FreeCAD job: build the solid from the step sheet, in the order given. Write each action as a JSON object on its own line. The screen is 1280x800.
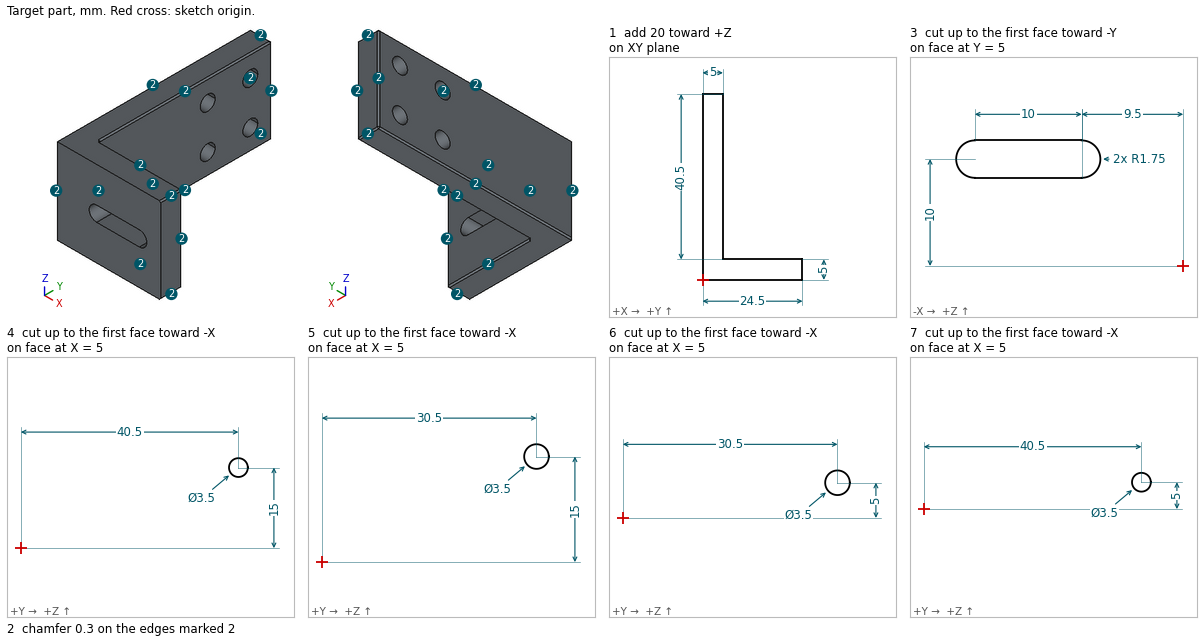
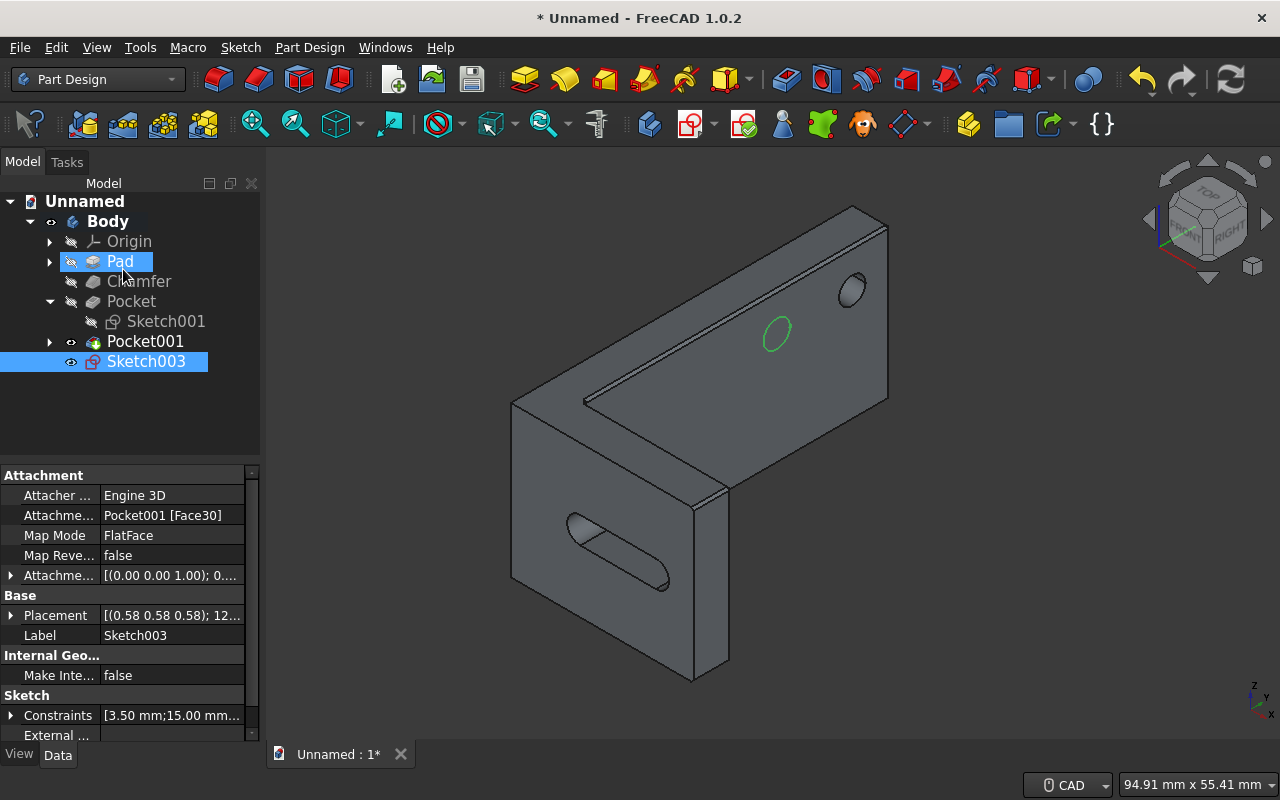
{"action": "left_click", "coordinate": [788, 80]}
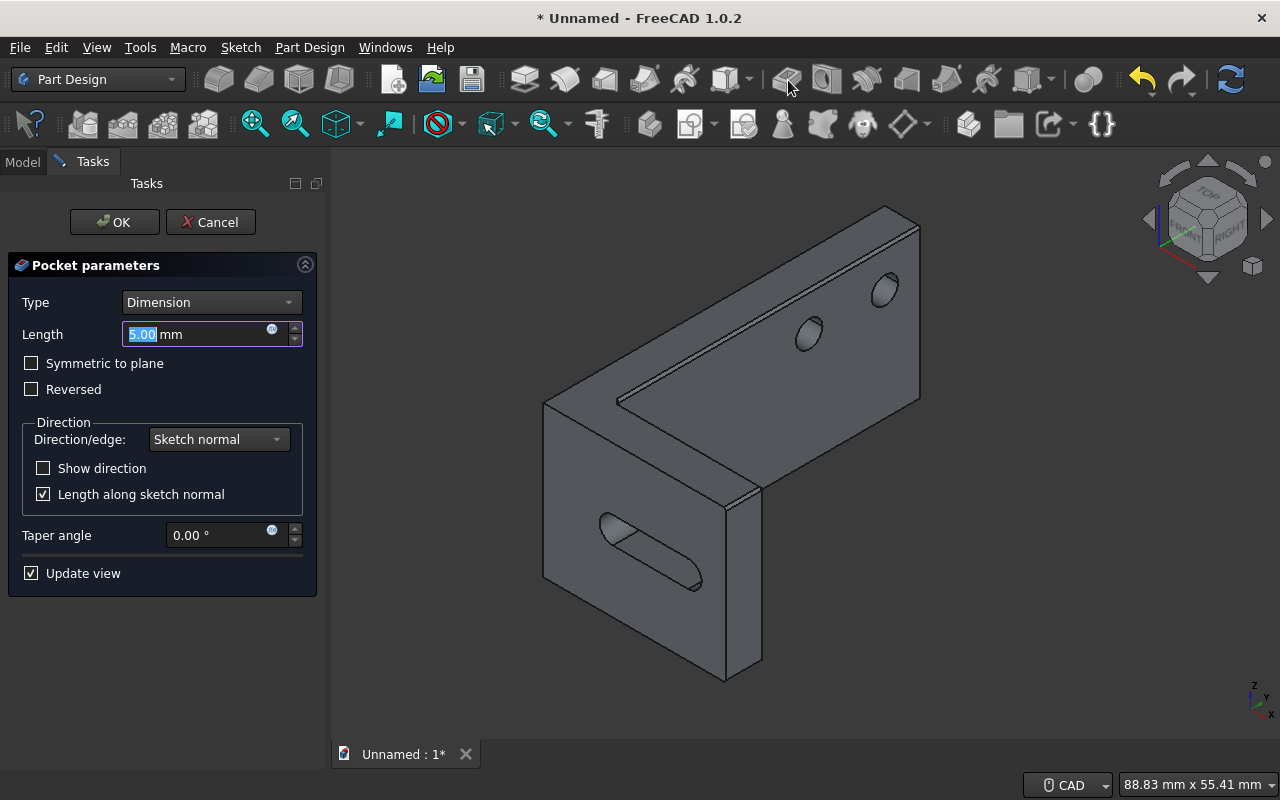
{"action": "left_click", "coordinate": [212, 302]}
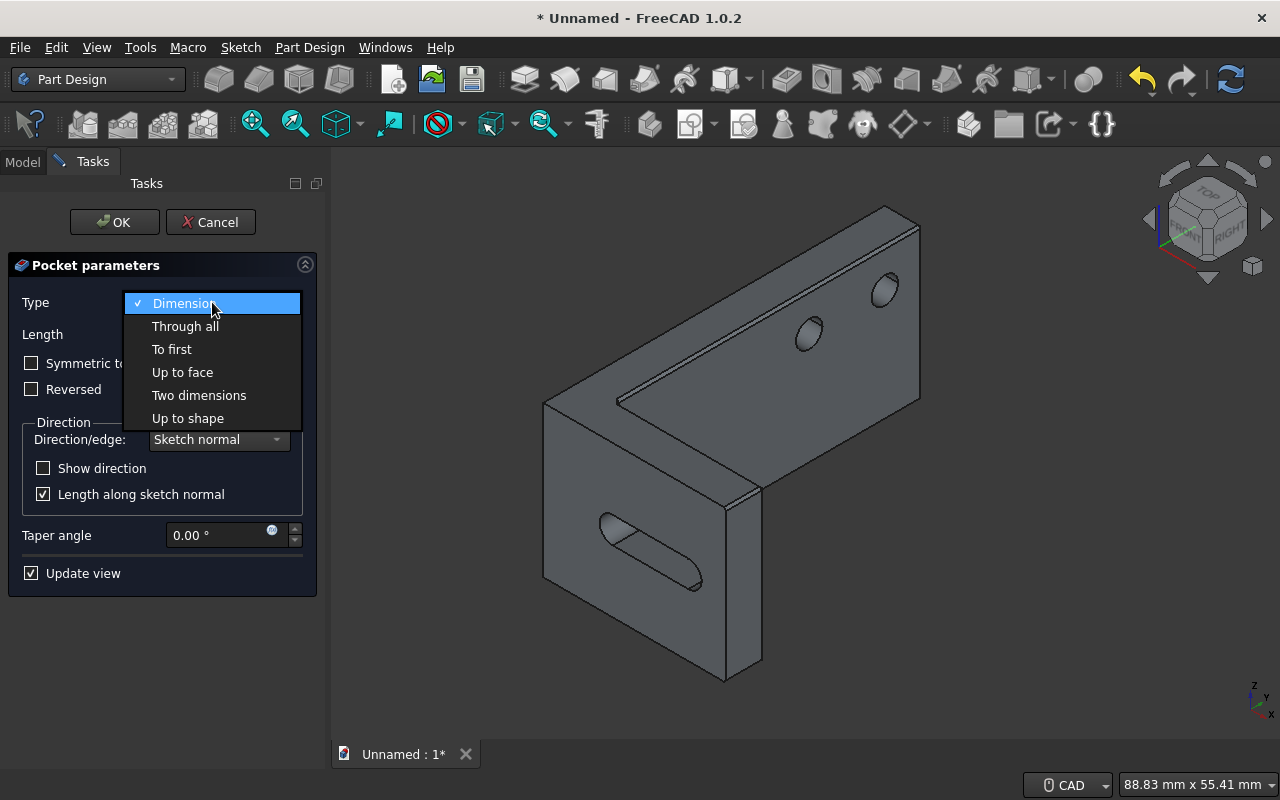
{"action": "left_click", "coordinate": [212, 350]}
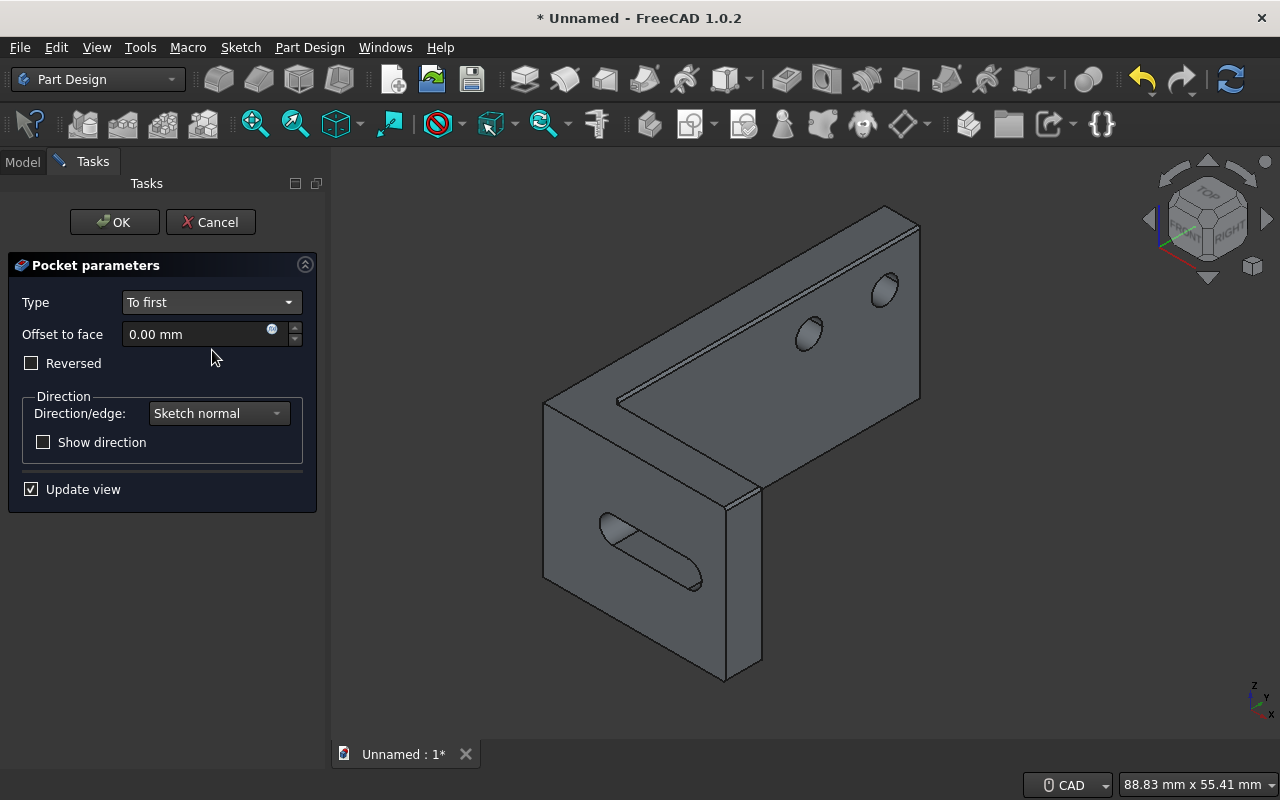
{"action": "left_click", "coordinate": [115, 222]}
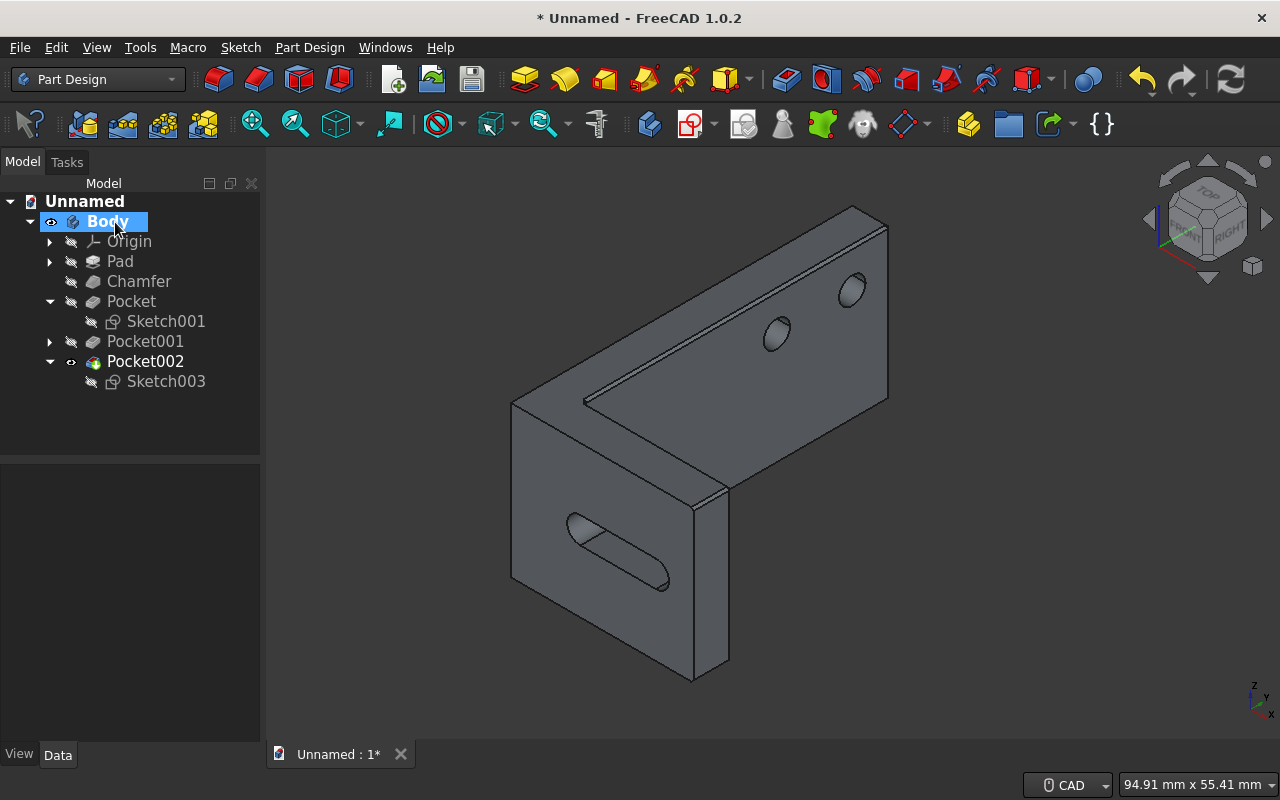
{"action": "left_click", "coordinate": [694, 424]}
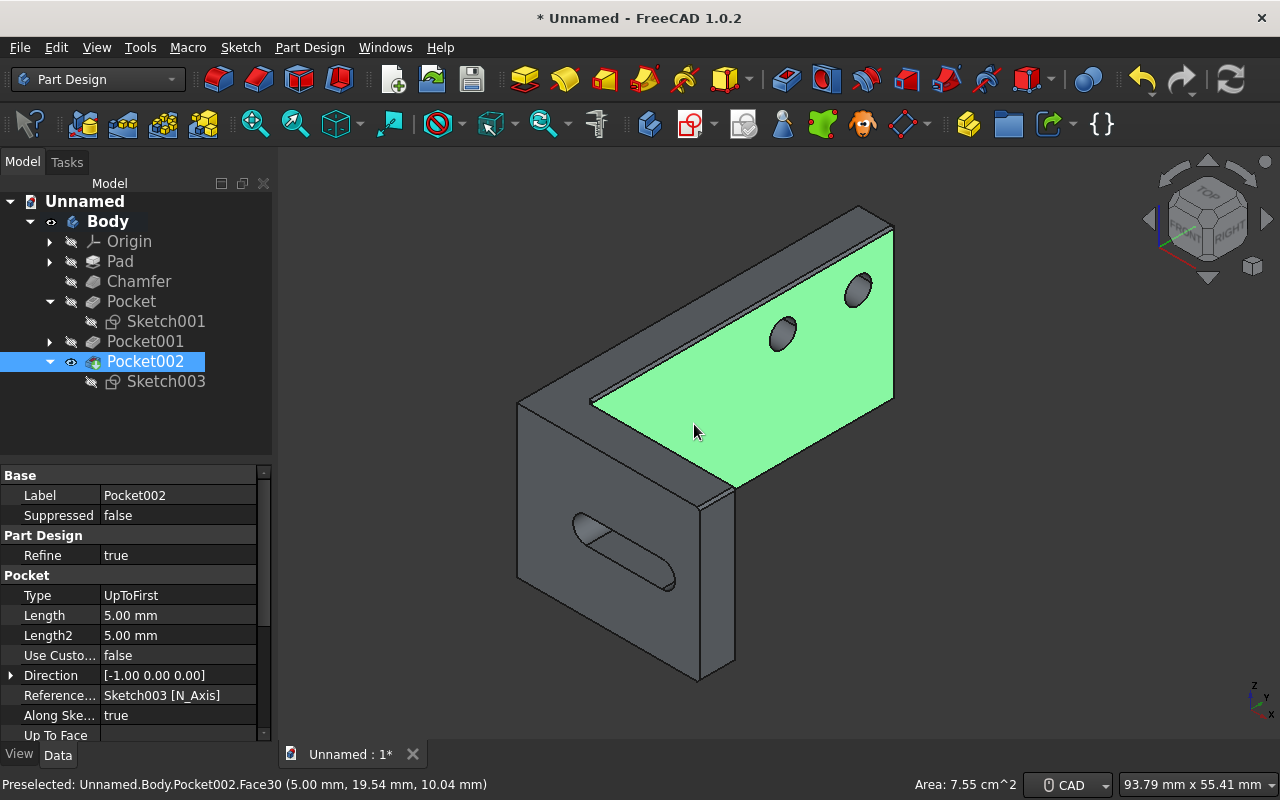
{"action": "left_click", "coordinate": [690, 124]}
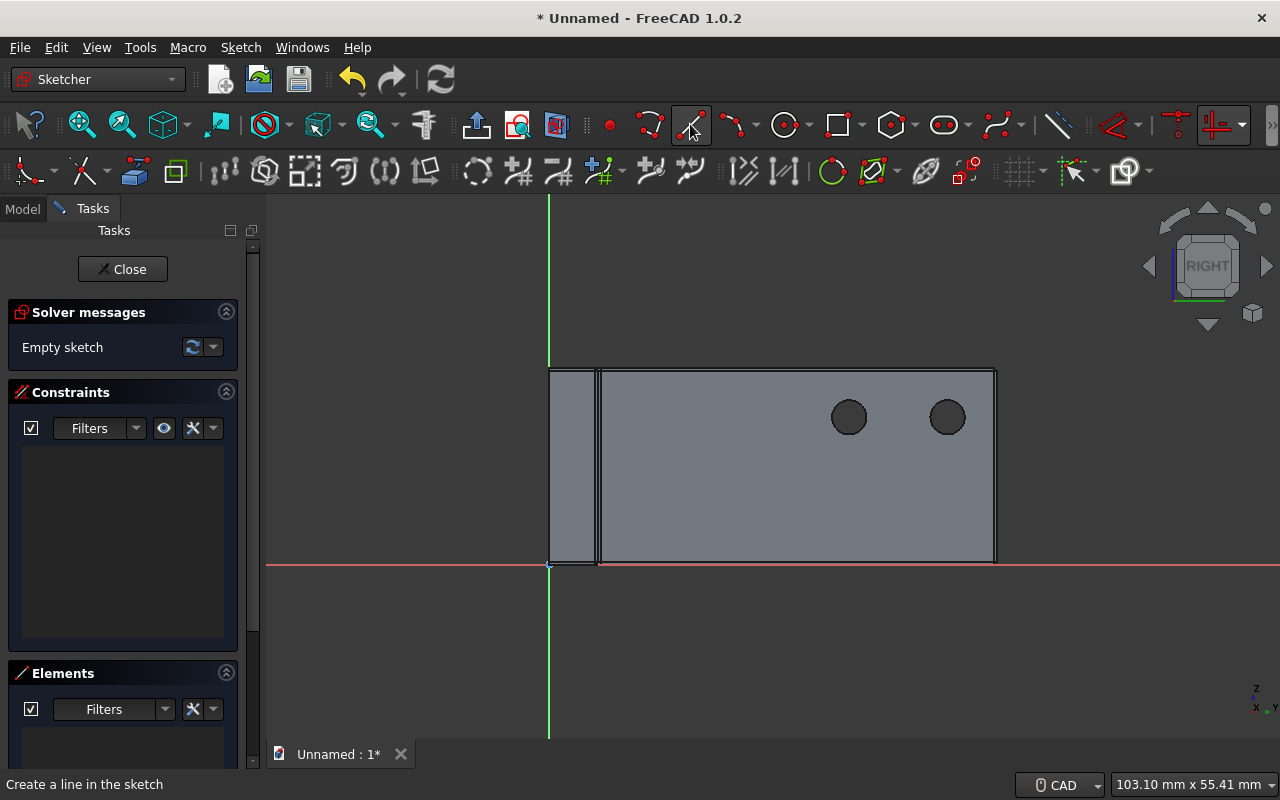
{"action": "left_click", "coordinate": [558, 126]}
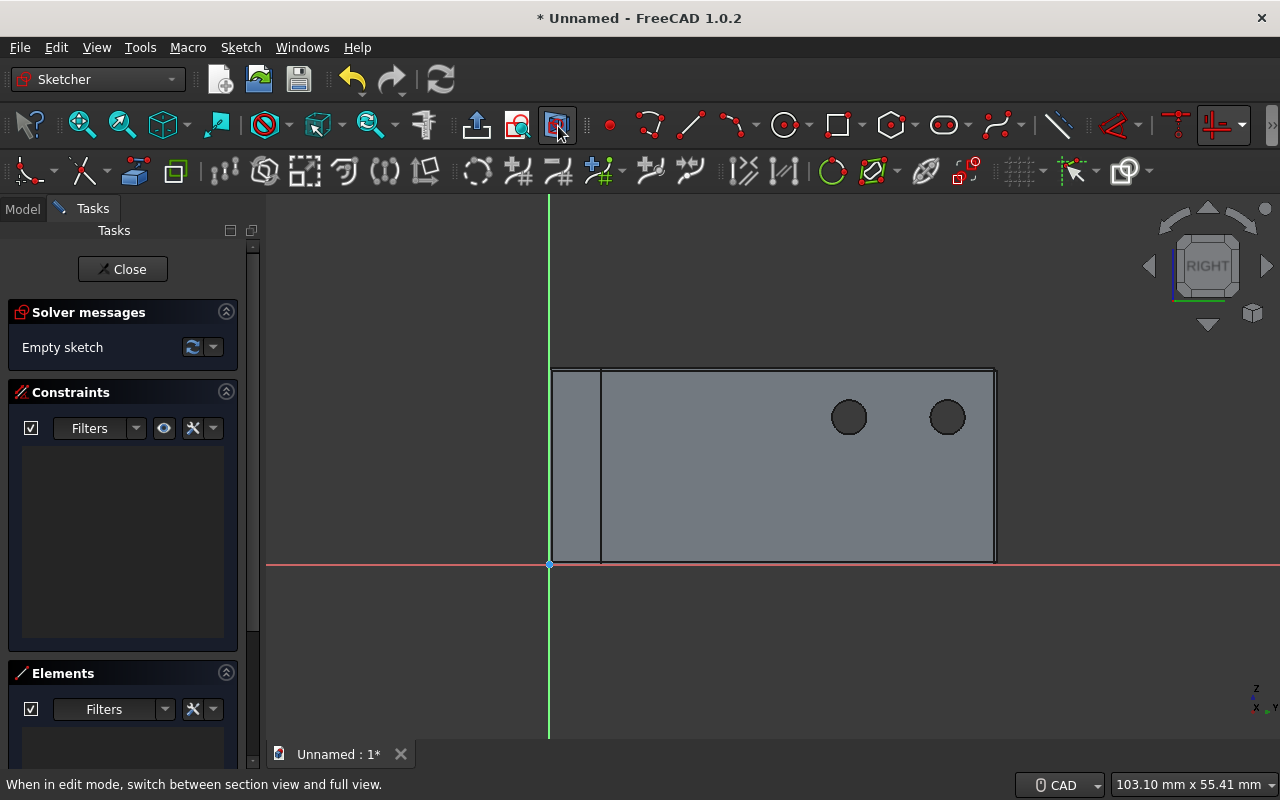
{"action": "scroll", "coordinate": [864, 521], "scroll_direction": "up", "scroll_amount": 12}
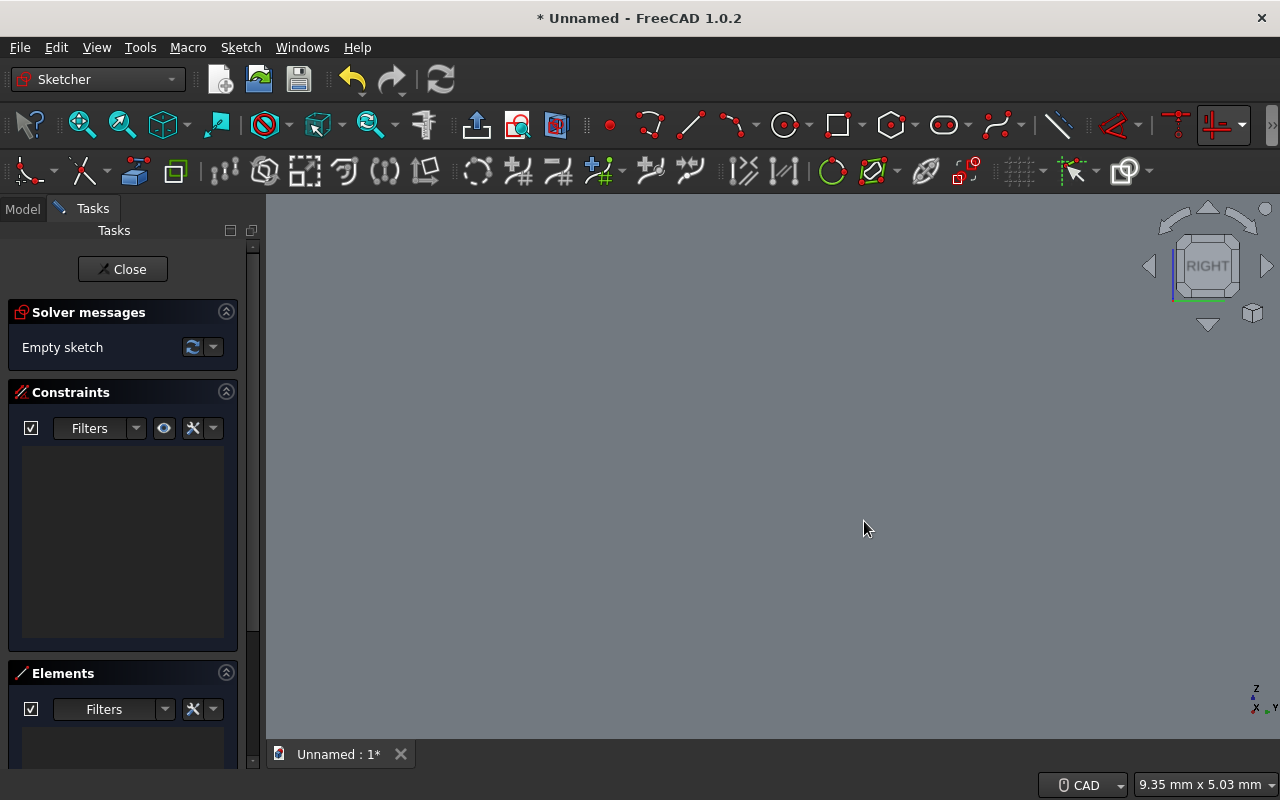
{"action": "left_click", "coordinate": [786, 126]}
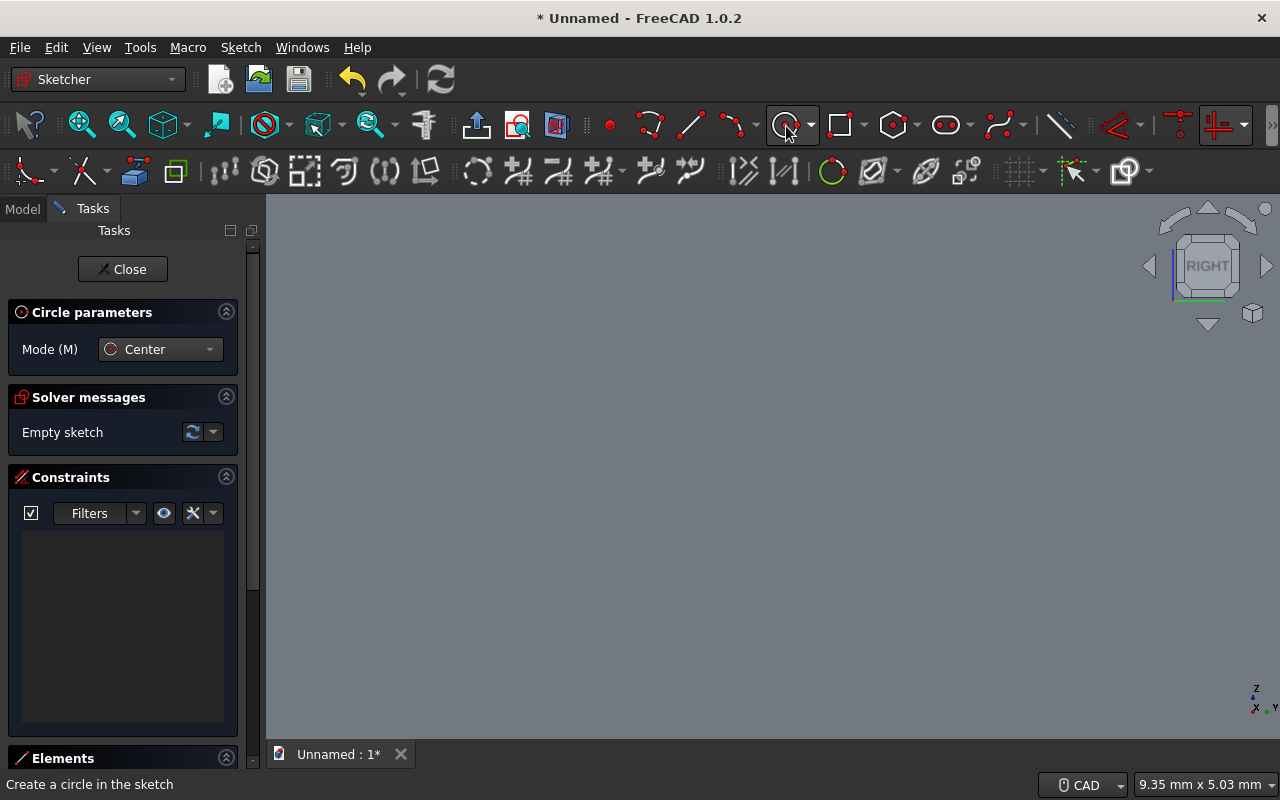
{"action": "left_click", "coordinate": [695, 456]}
{"action": "left_click", "coordinate": [829, 322]}
{"action": "key", "text": "Escape"}